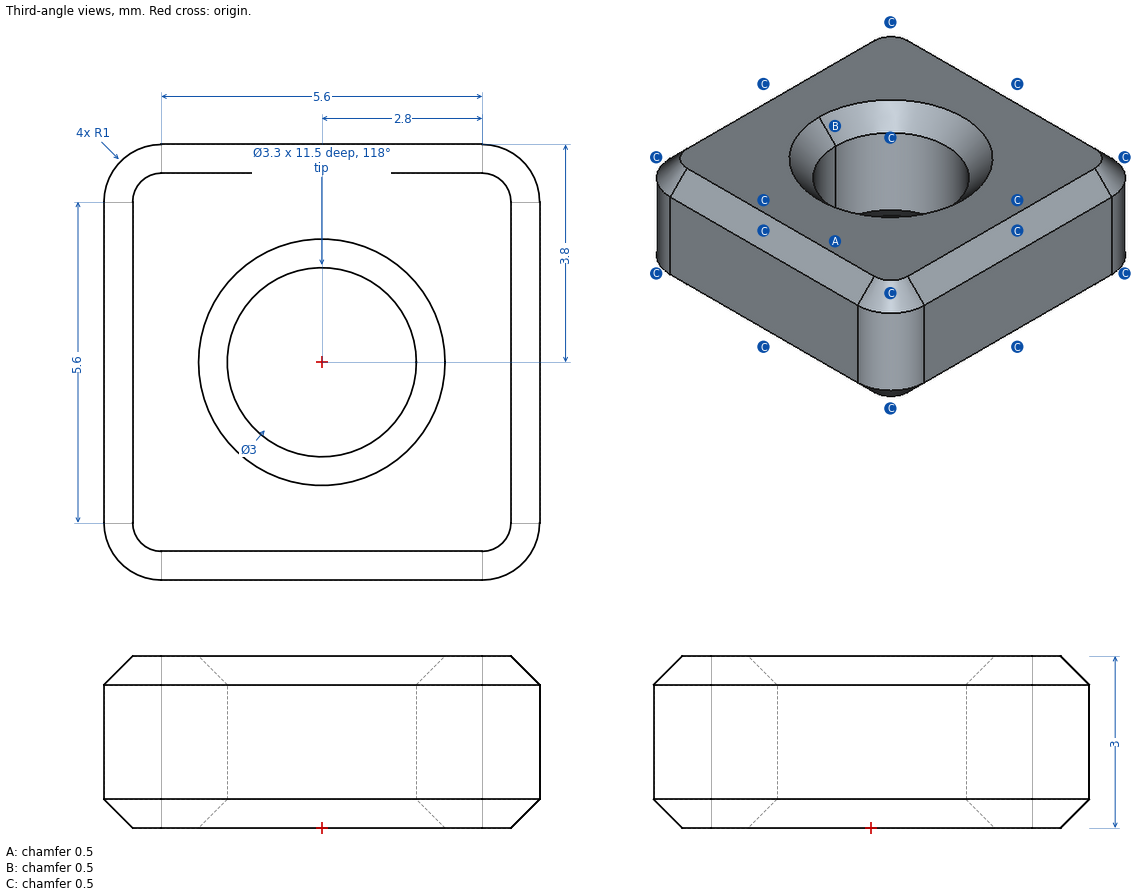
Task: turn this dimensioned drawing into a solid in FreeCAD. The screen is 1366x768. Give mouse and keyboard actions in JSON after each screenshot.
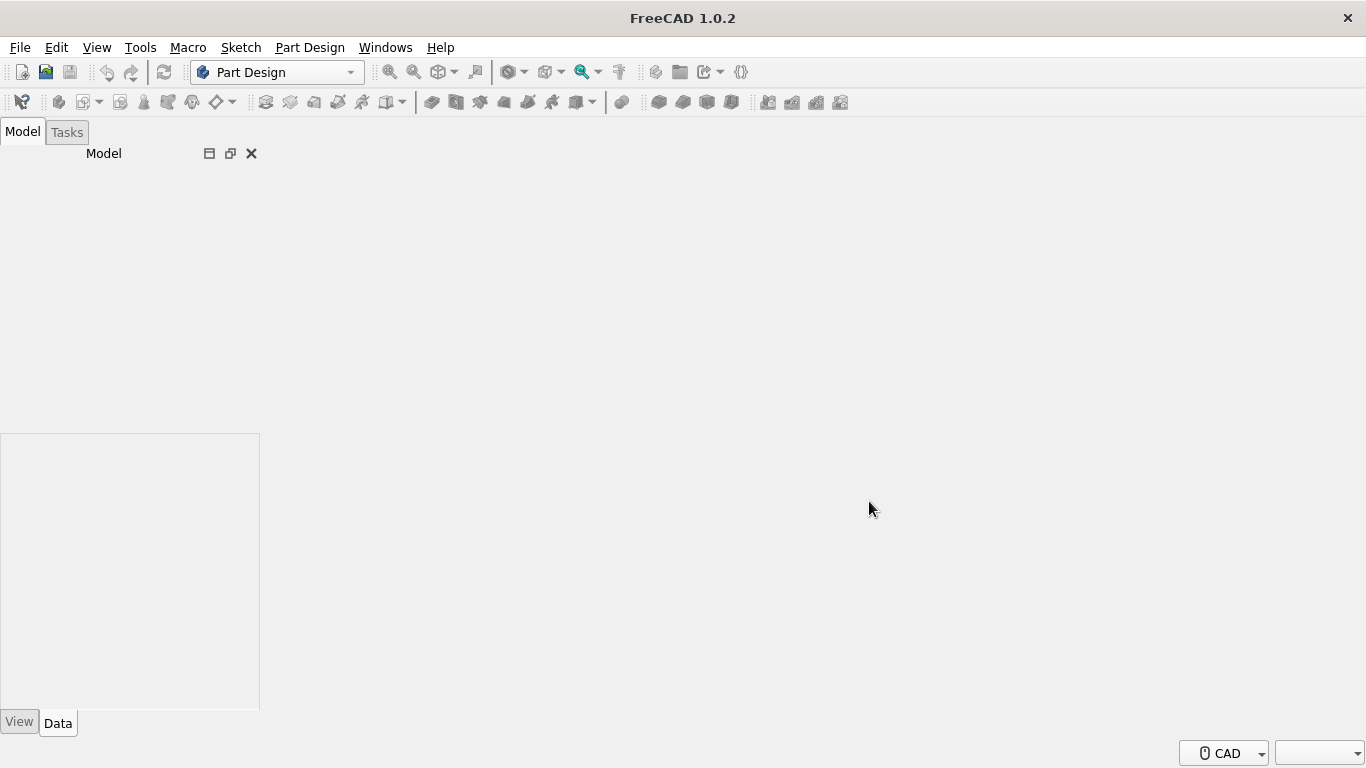
{"action": "key", "text": "ctrl+n"}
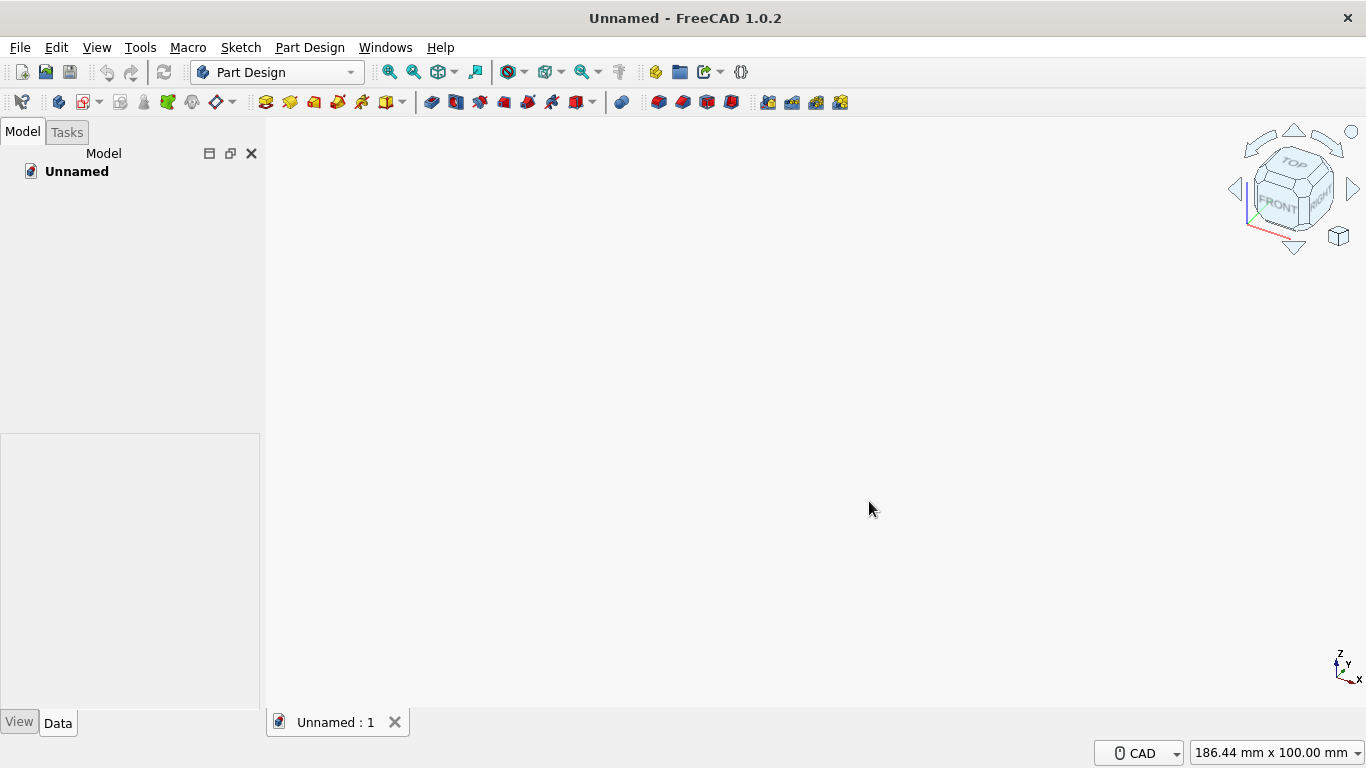
{"action": "left_click", "coordinate": [84, 102]}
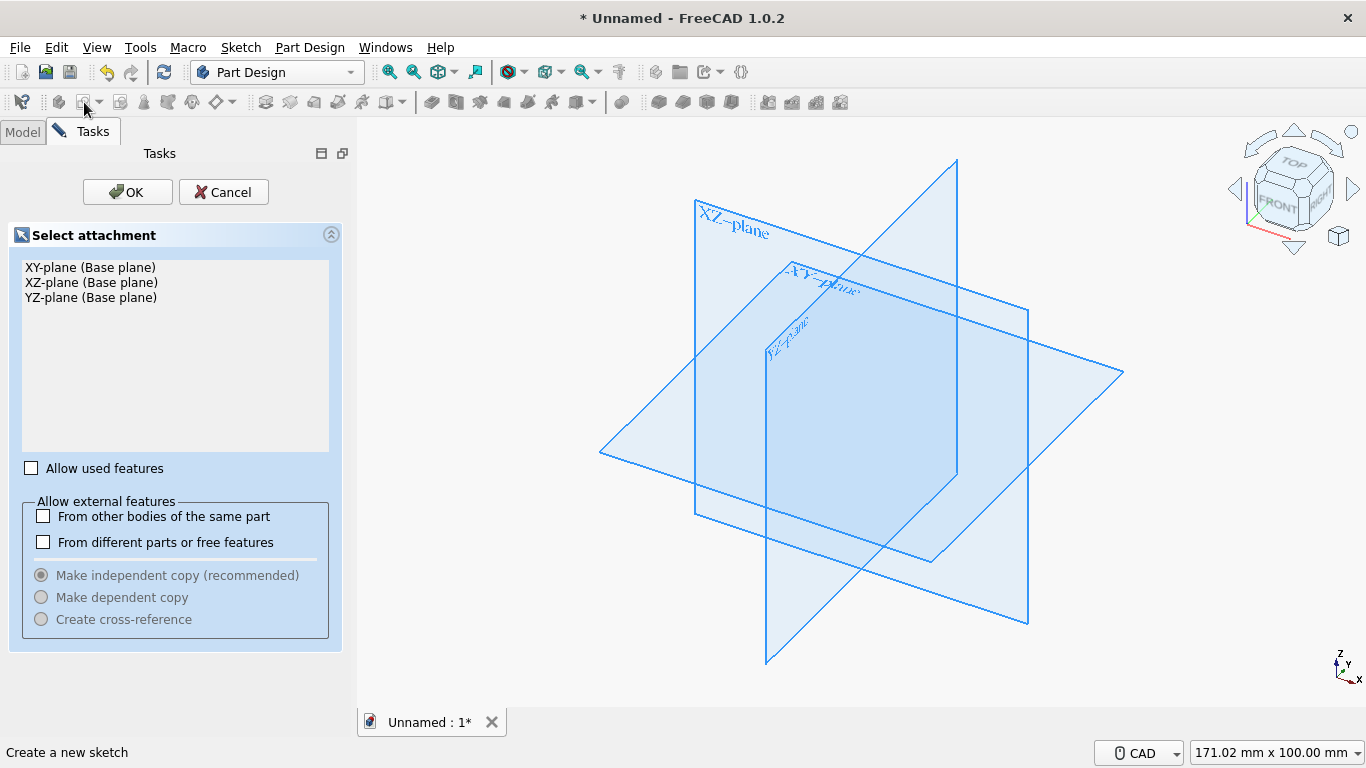
{"action": "left_click", "coordinate": [82, 268]}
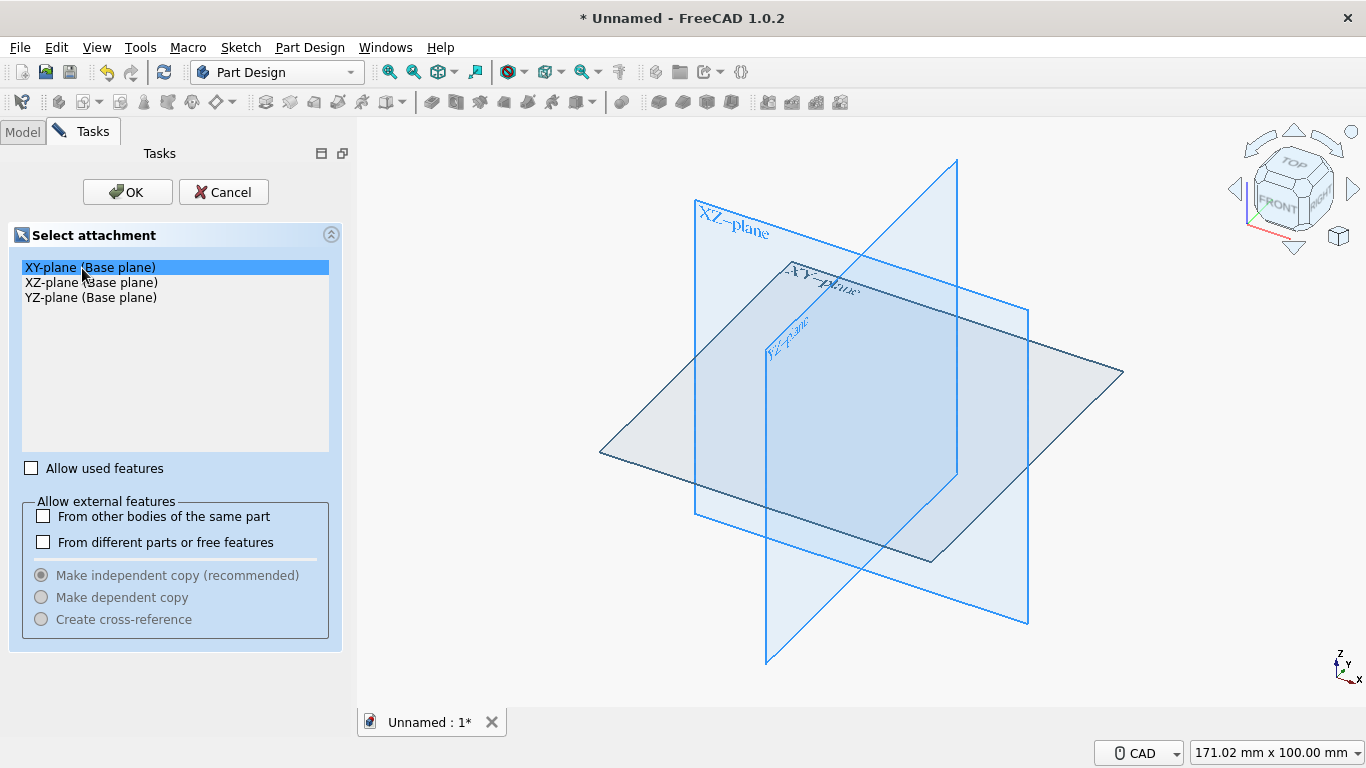
{"action": "left_click", "coordinate": [128, 192]}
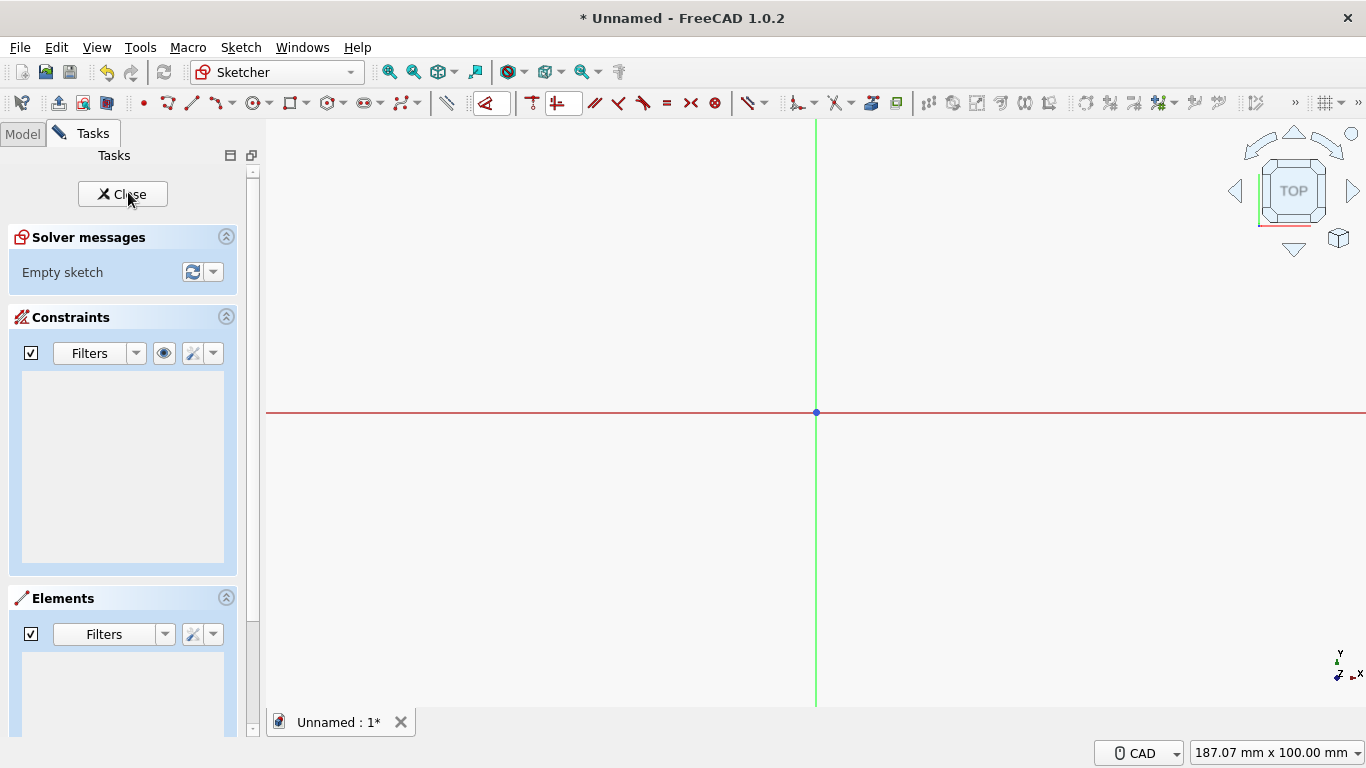
{"action": "scroll", "coordinate": [825, 413], "scroll_direction": "up", "scroll_amount": 11}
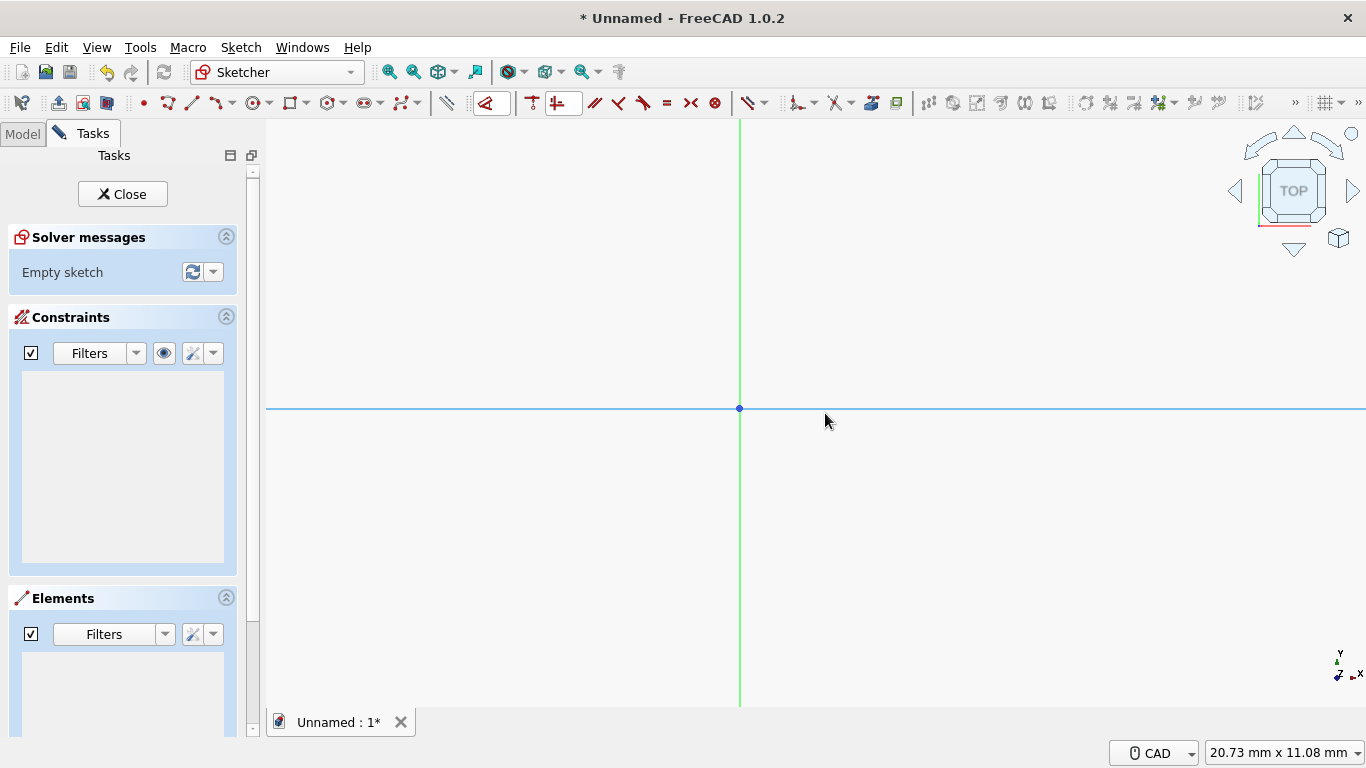
{"action": "key", "text": "g l"}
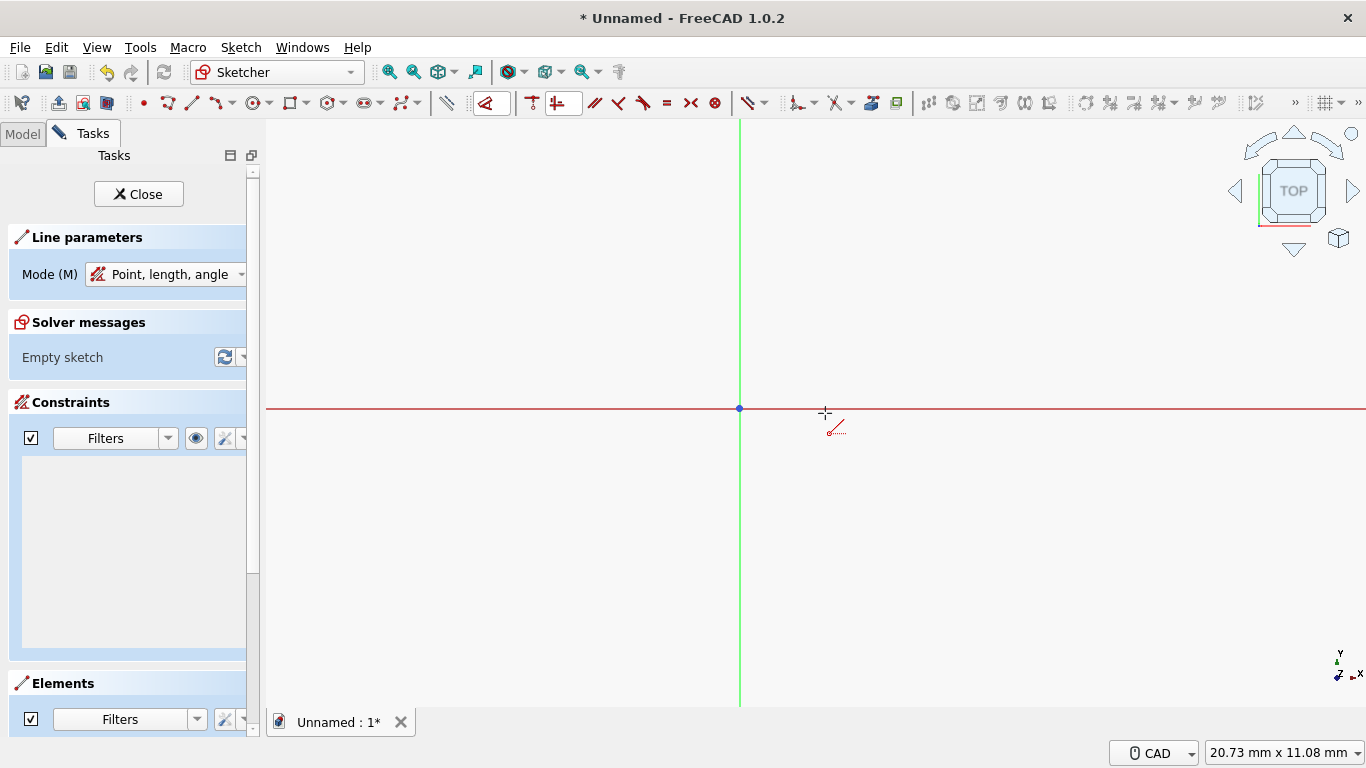
{"action": "left_click", "coordinate": [888, 207]}
{"action": "left_click", "coordinate": [591, 207]}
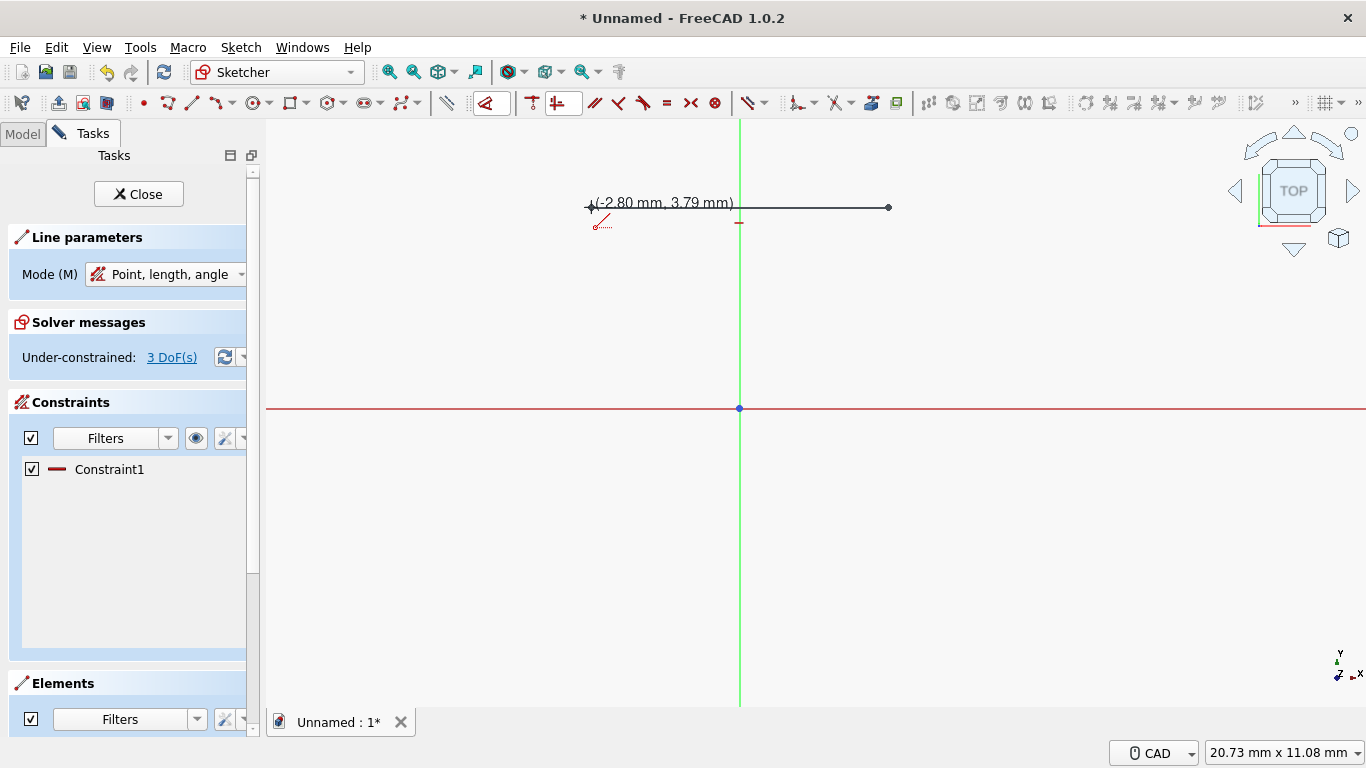
{"action": "left_click", "coordinate": [538, 260]}
{"action": "left_click", "coordinate": [538, 558]}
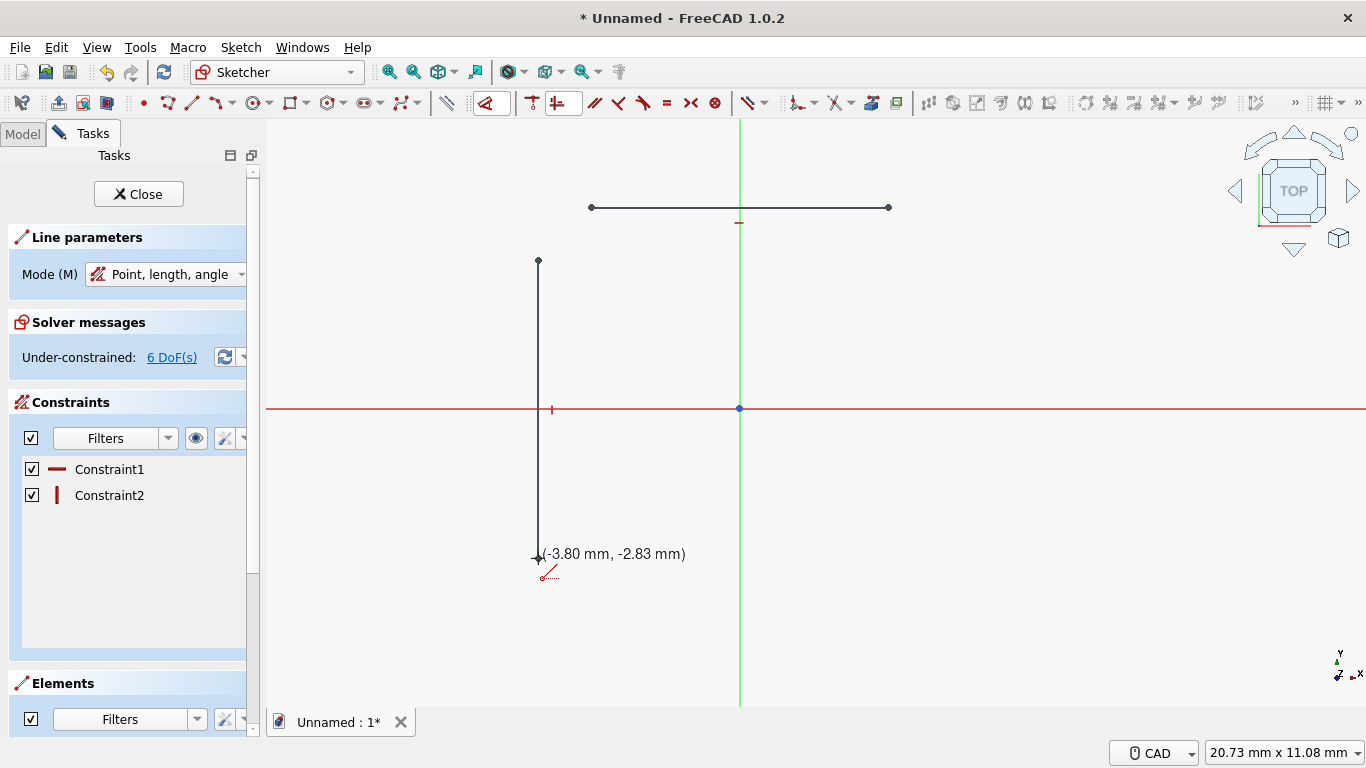
{"action": "left_click", "coordinate": [591, 611]}
{"action": "left_click", "coordinate": [888, 611]}